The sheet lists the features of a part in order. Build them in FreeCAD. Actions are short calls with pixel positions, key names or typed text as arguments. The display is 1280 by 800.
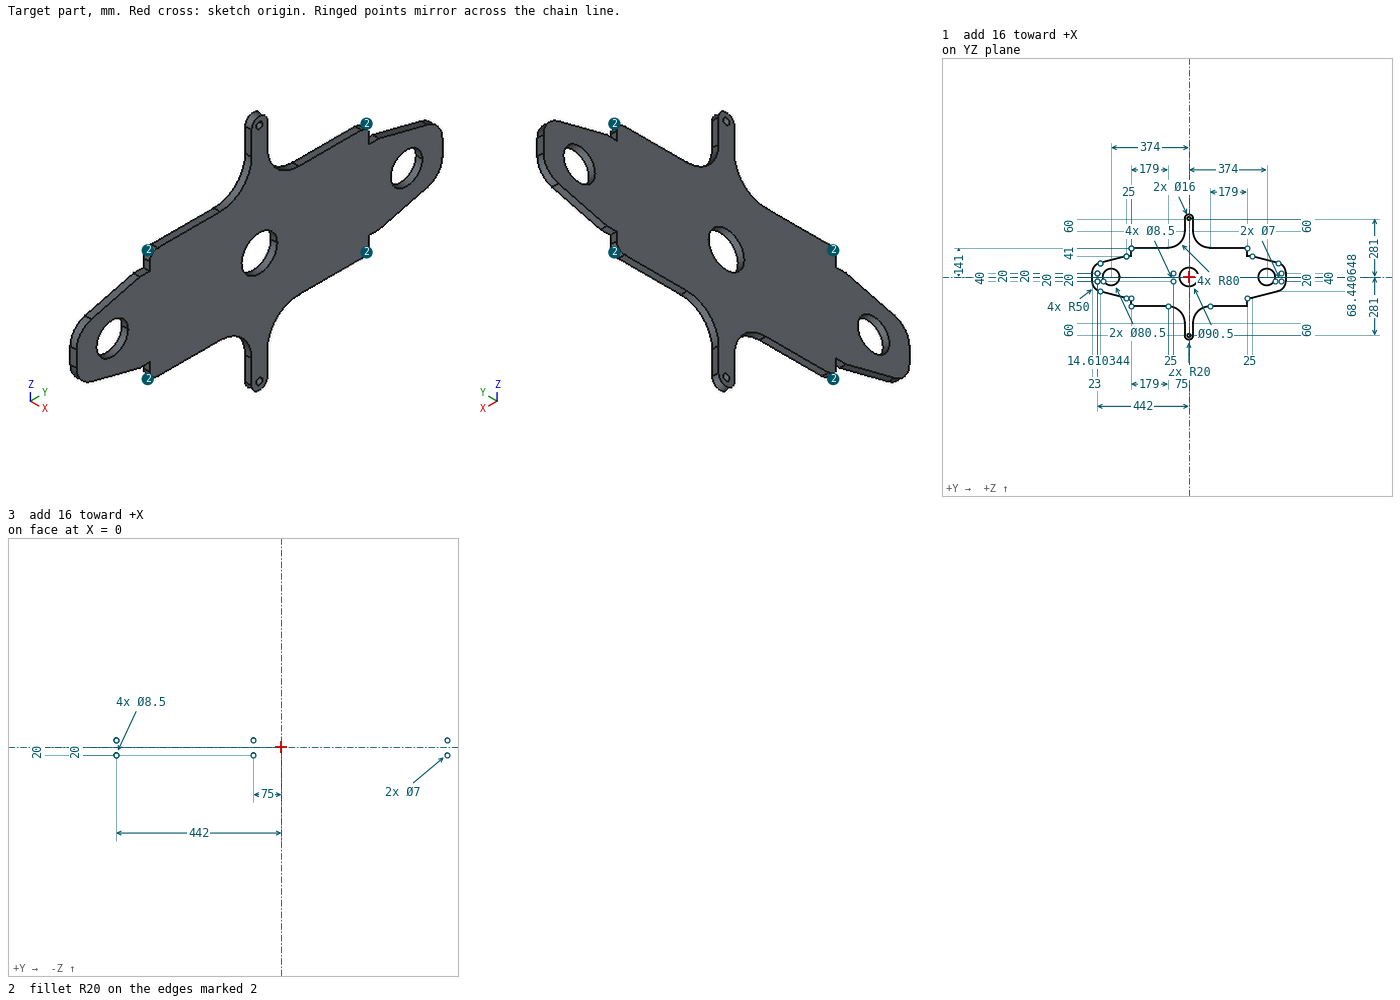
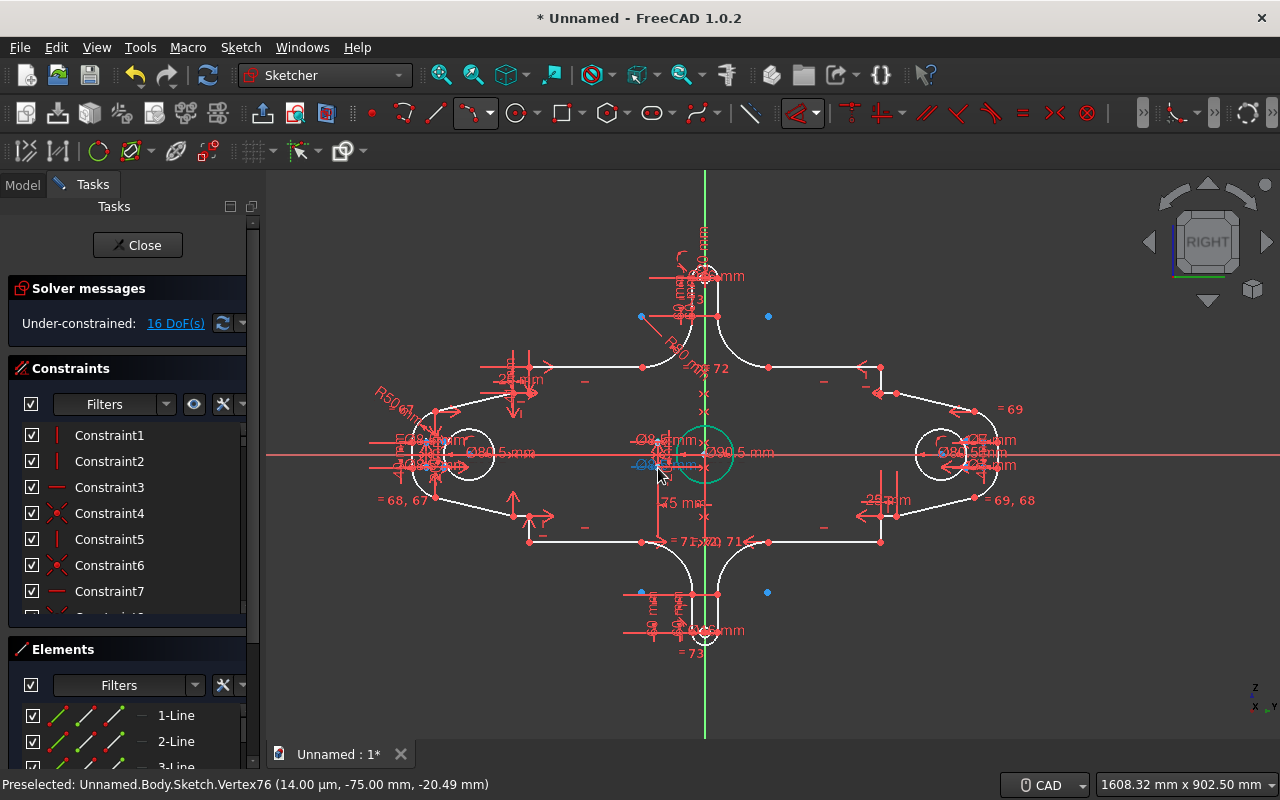
click(608, 367)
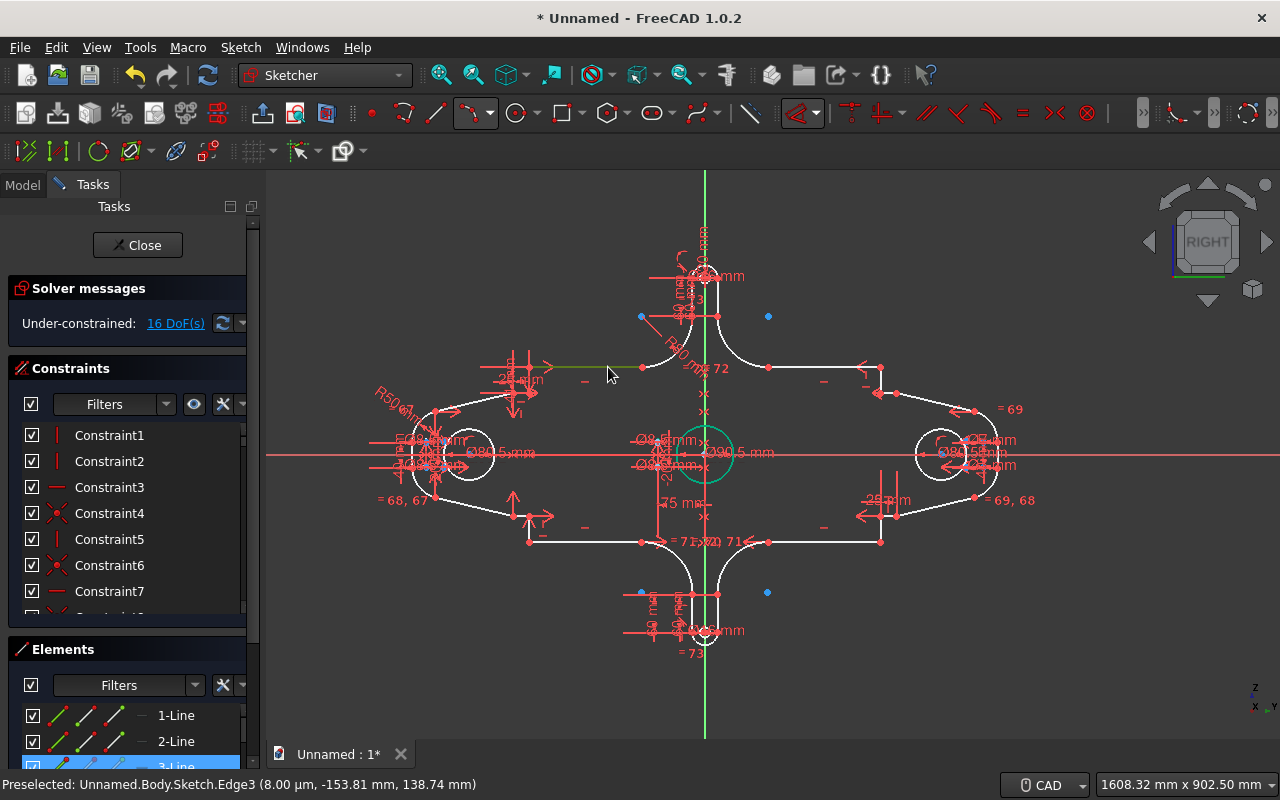
key(l)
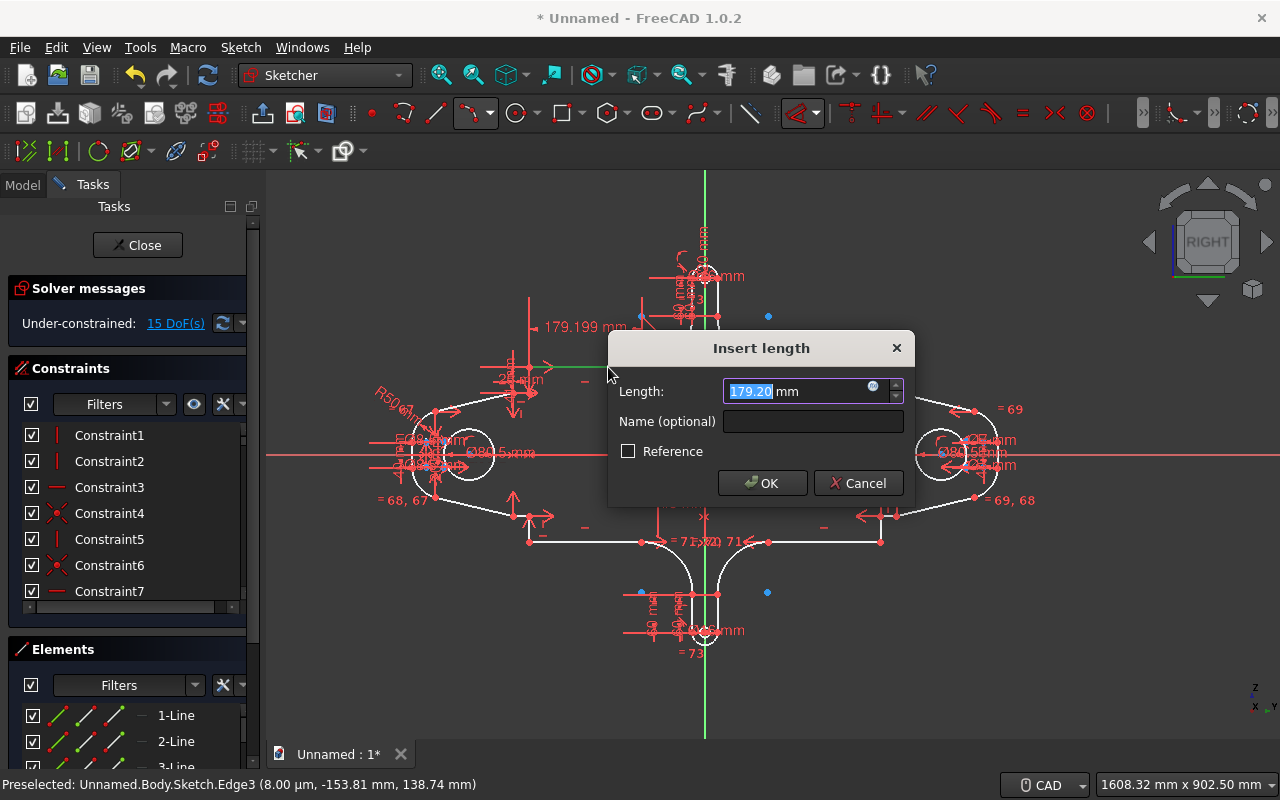
text(179)
key(Return)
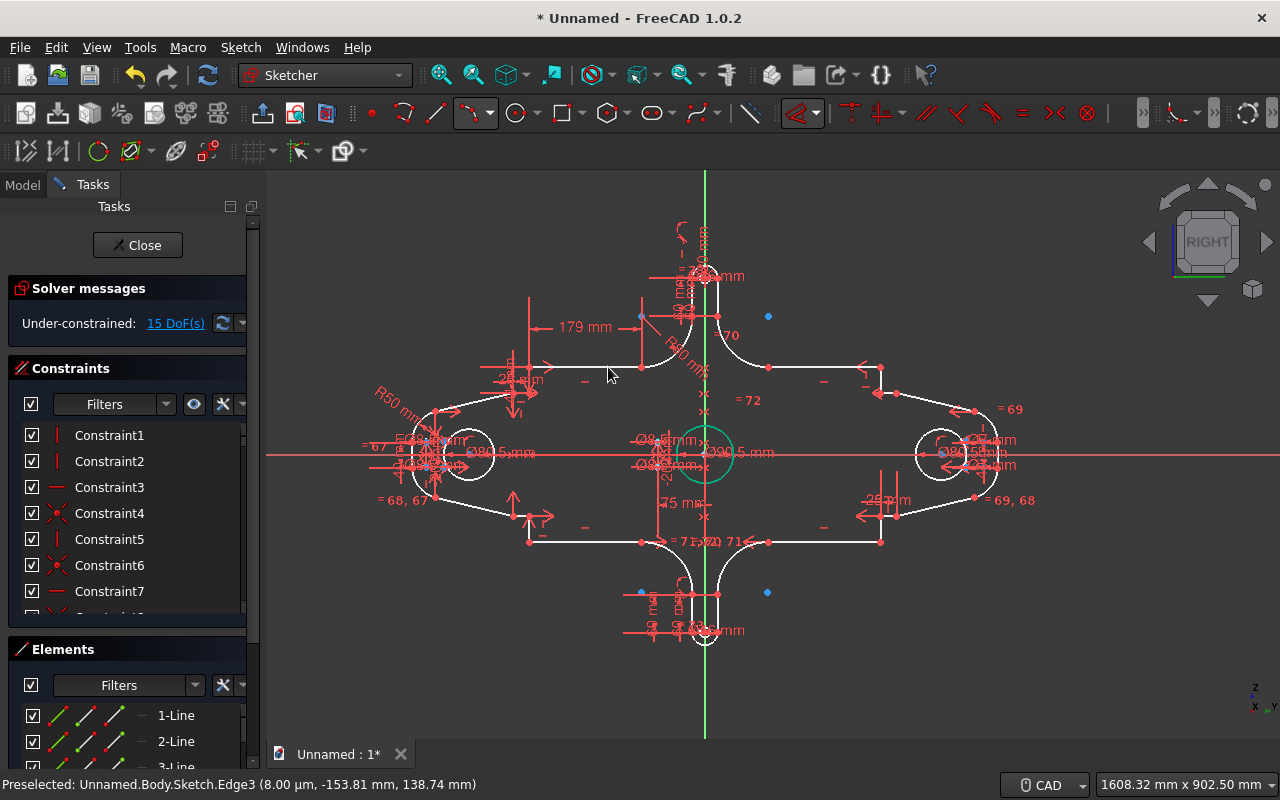
click(563, 542)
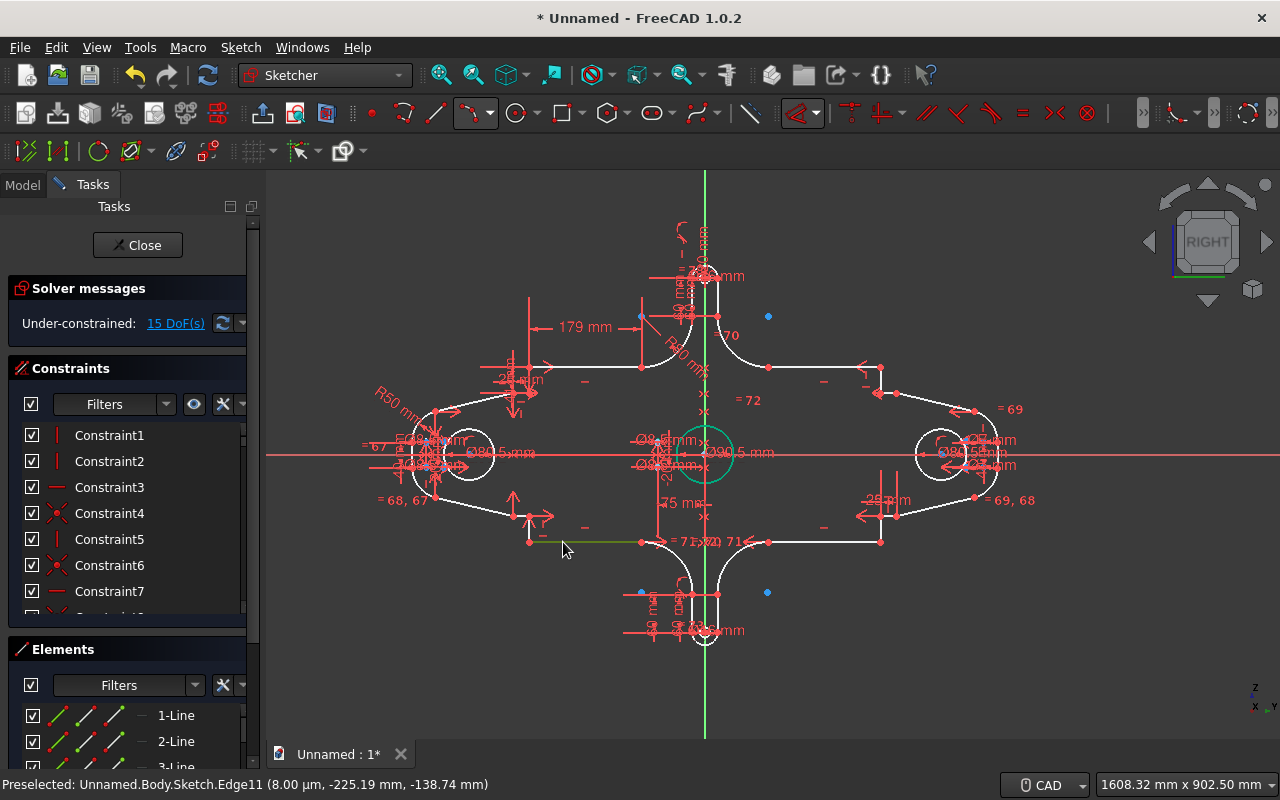
click(818, 114)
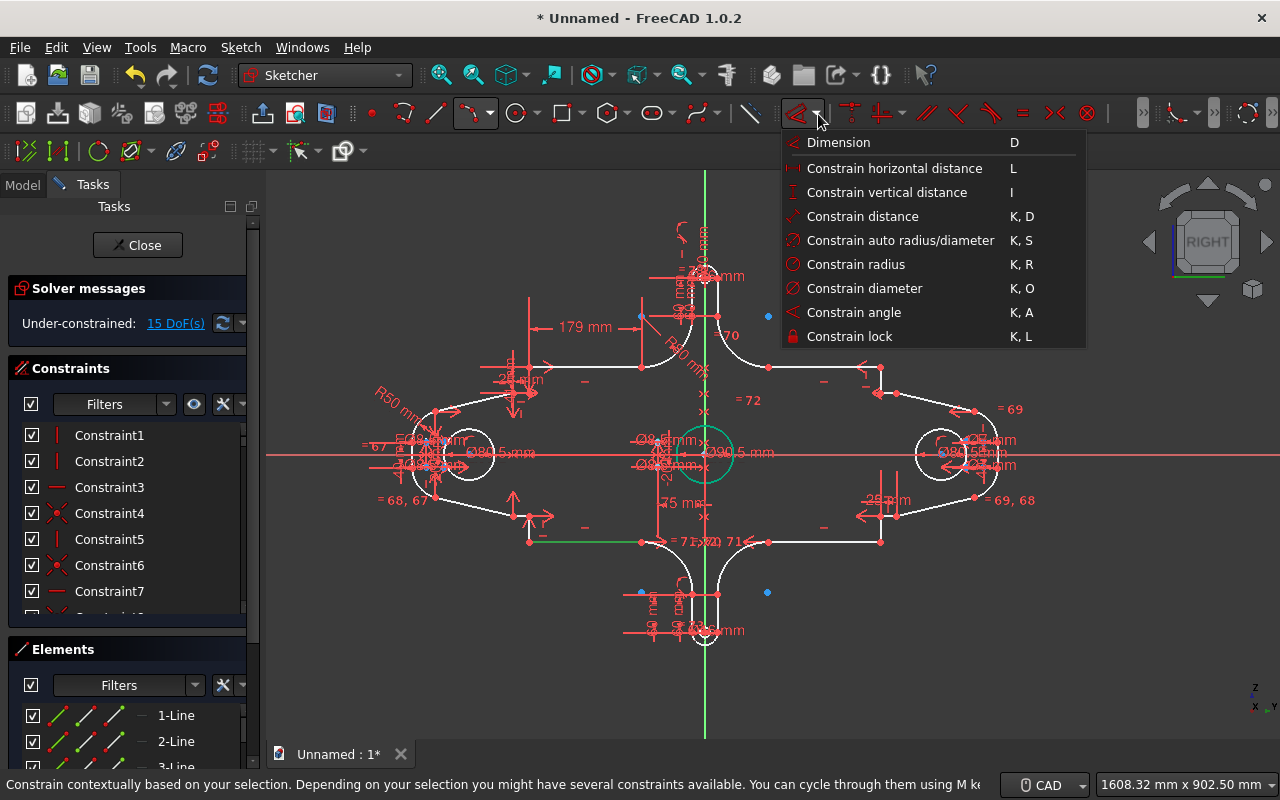
click(934, 168)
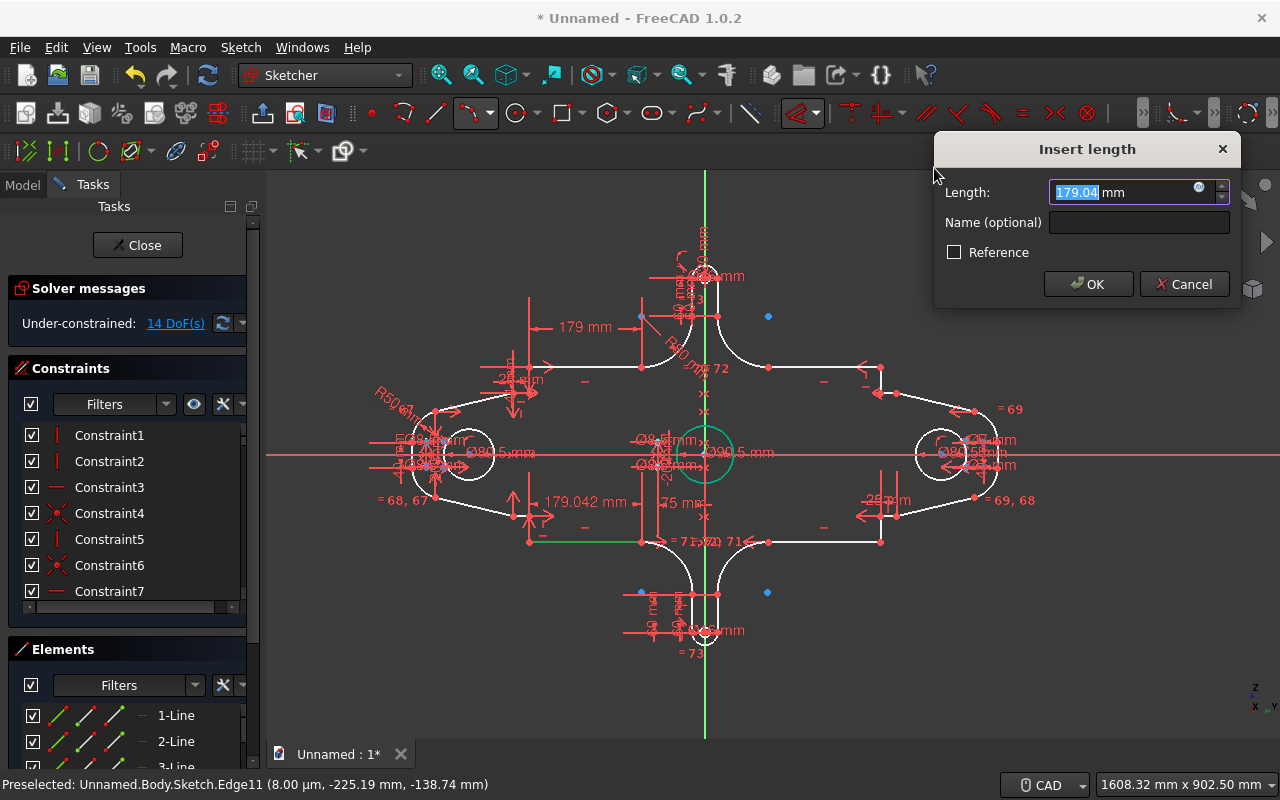
text(179)
key(Return)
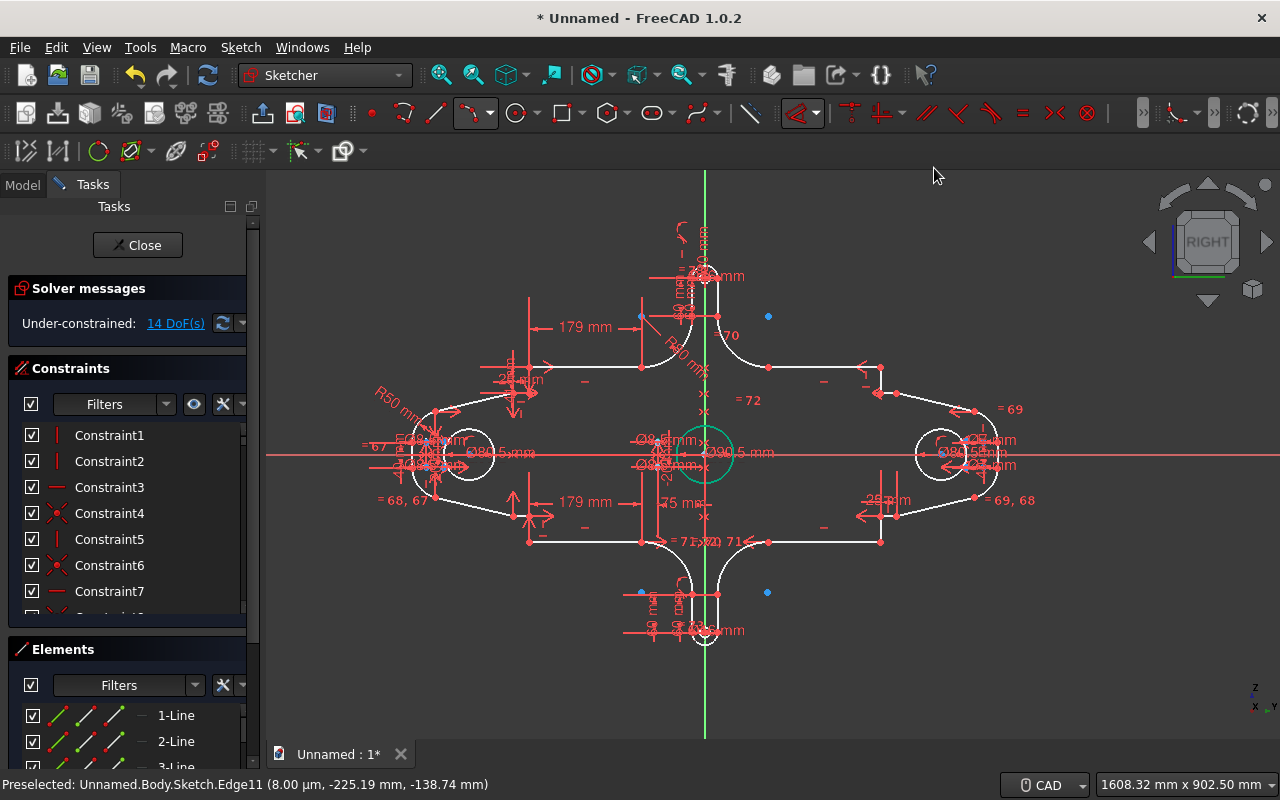
click(847, 367)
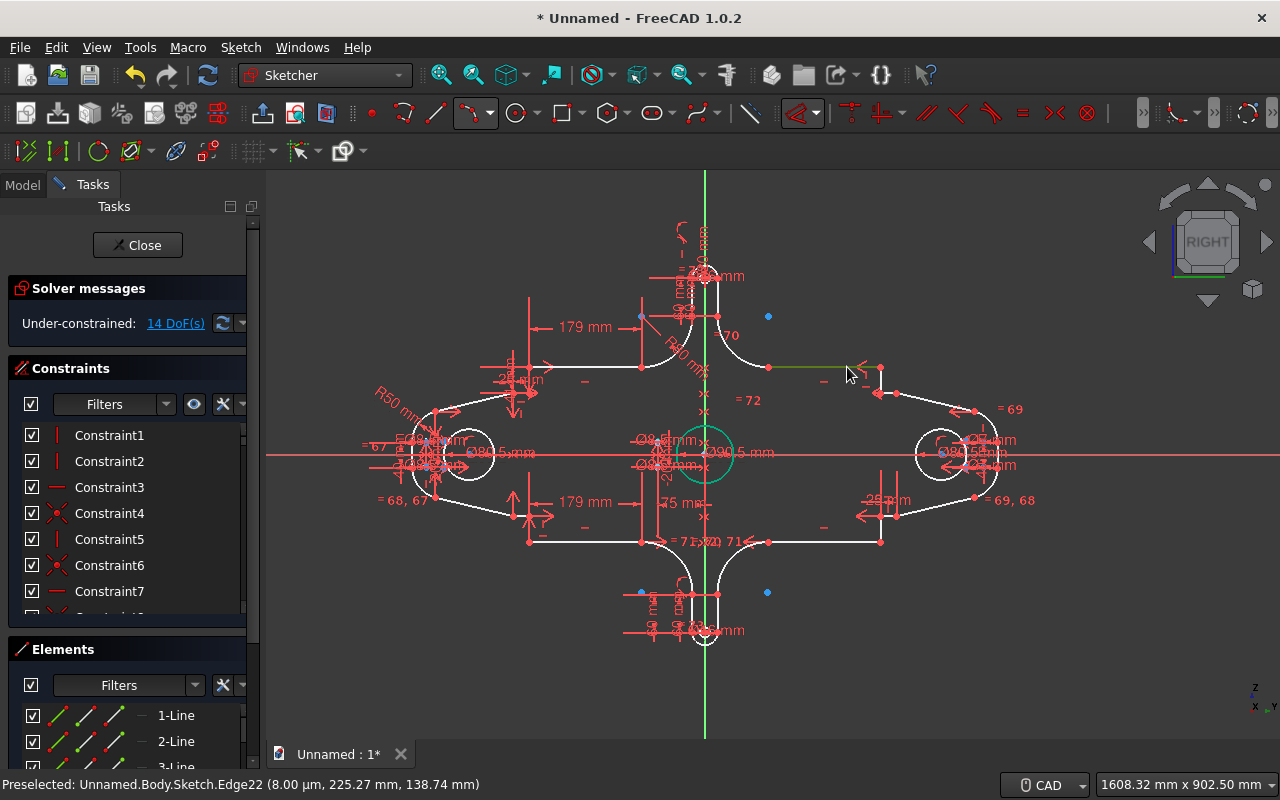
key(l)